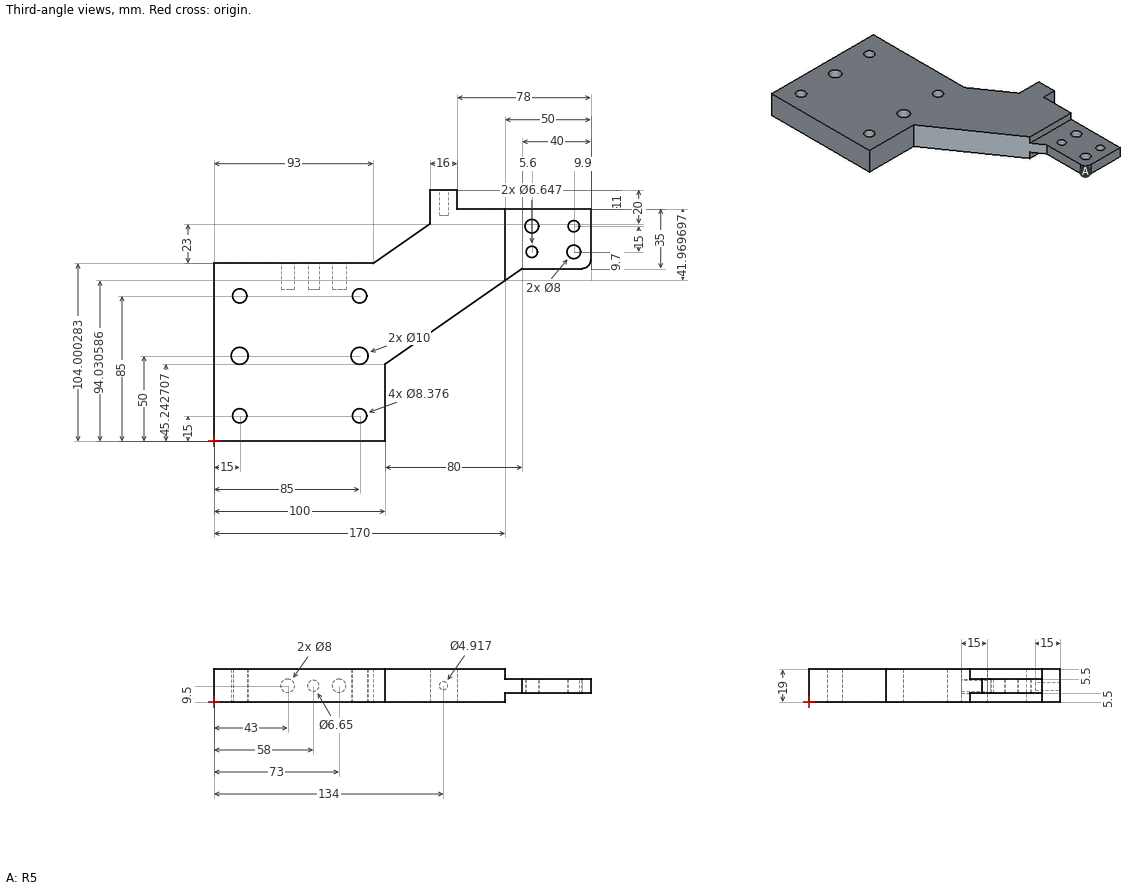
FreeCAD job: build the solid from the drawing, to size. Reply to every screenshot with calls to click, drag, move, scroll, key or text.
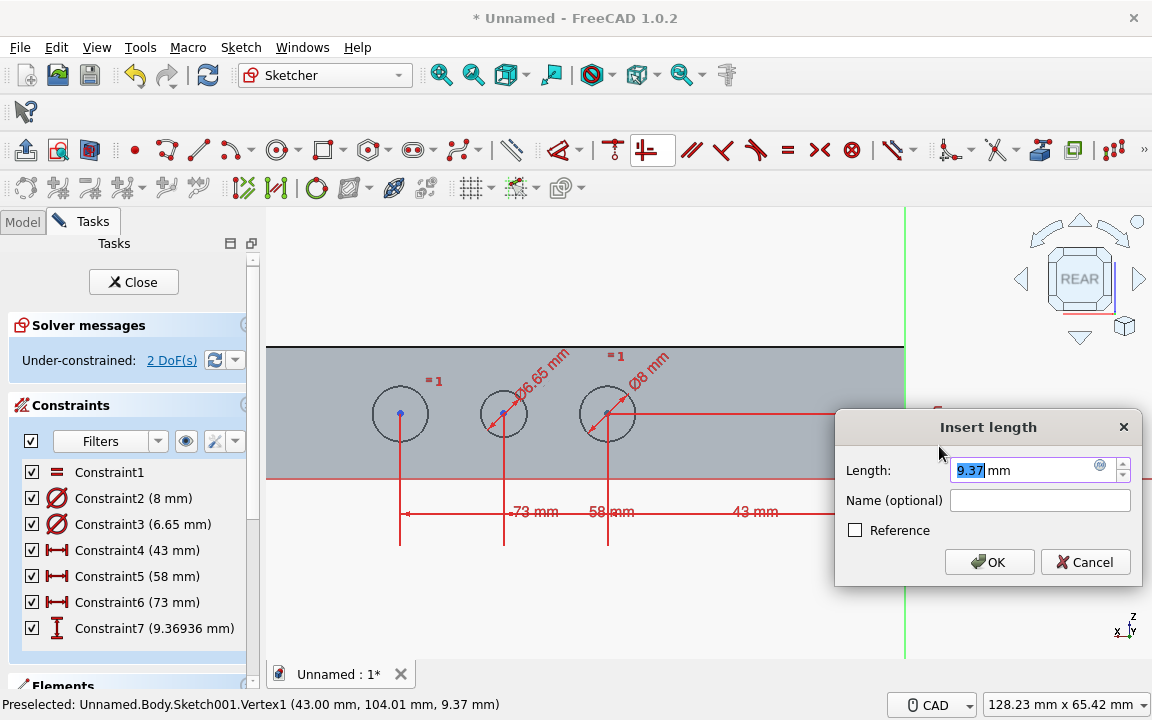
text(9.5)
key(Return)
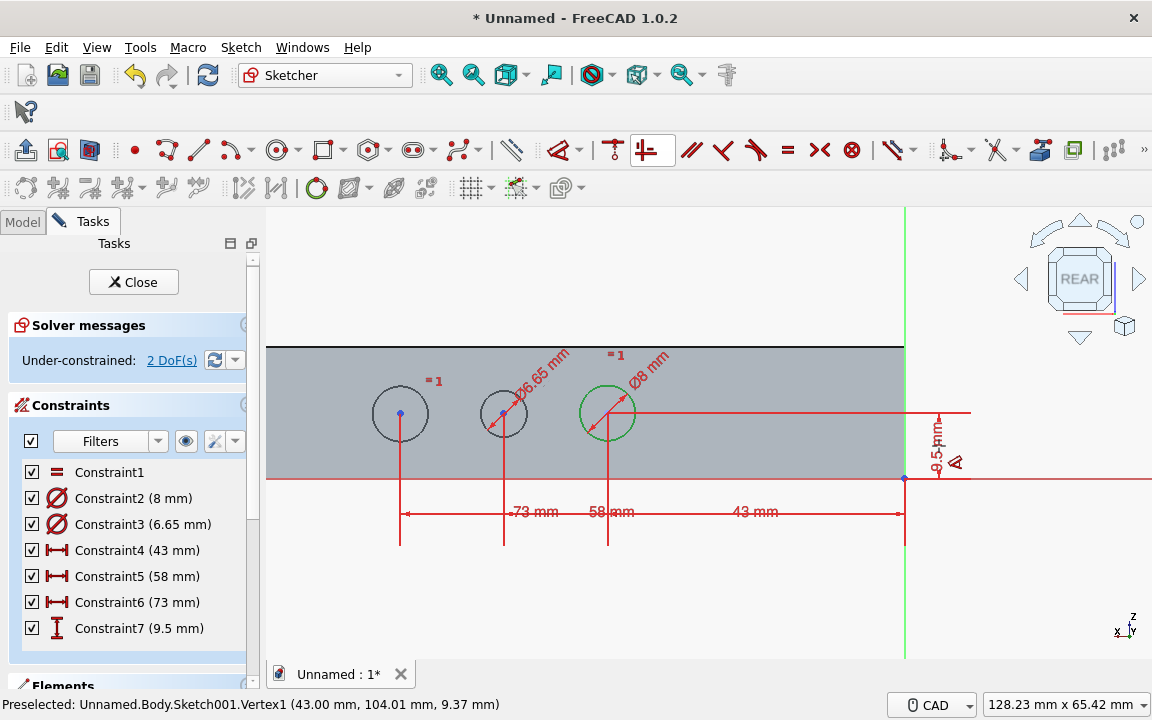
click(504, 414)
click(939, 424)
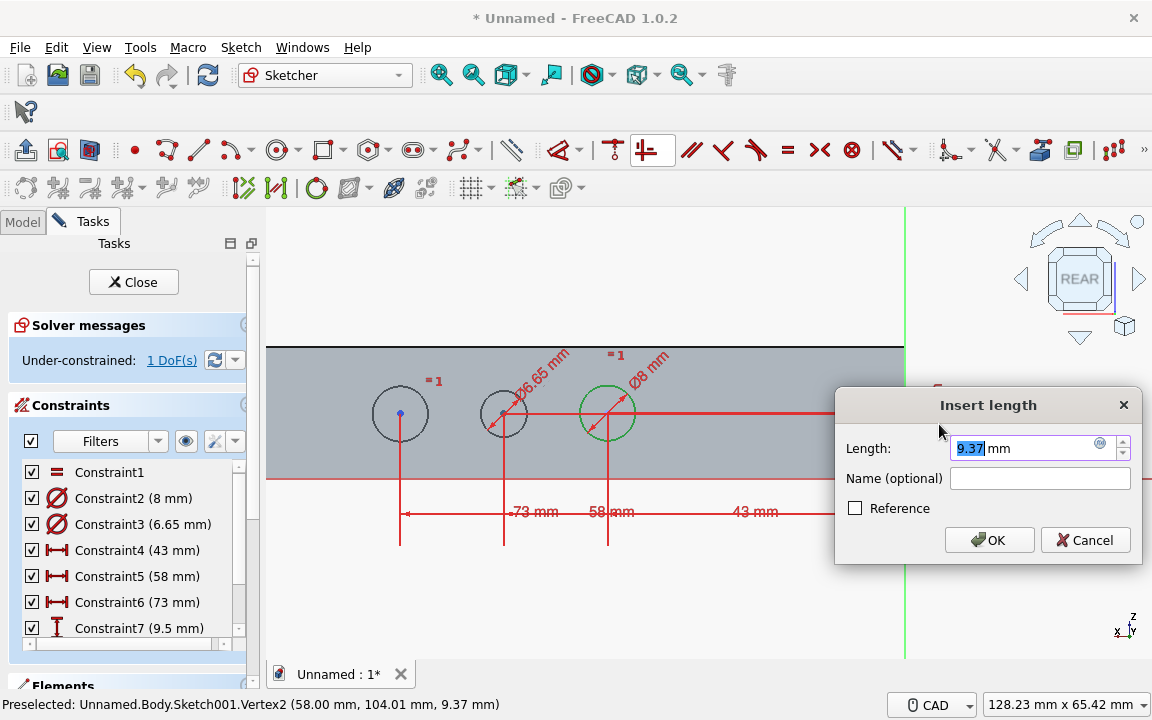
text(9.5)
key(Return)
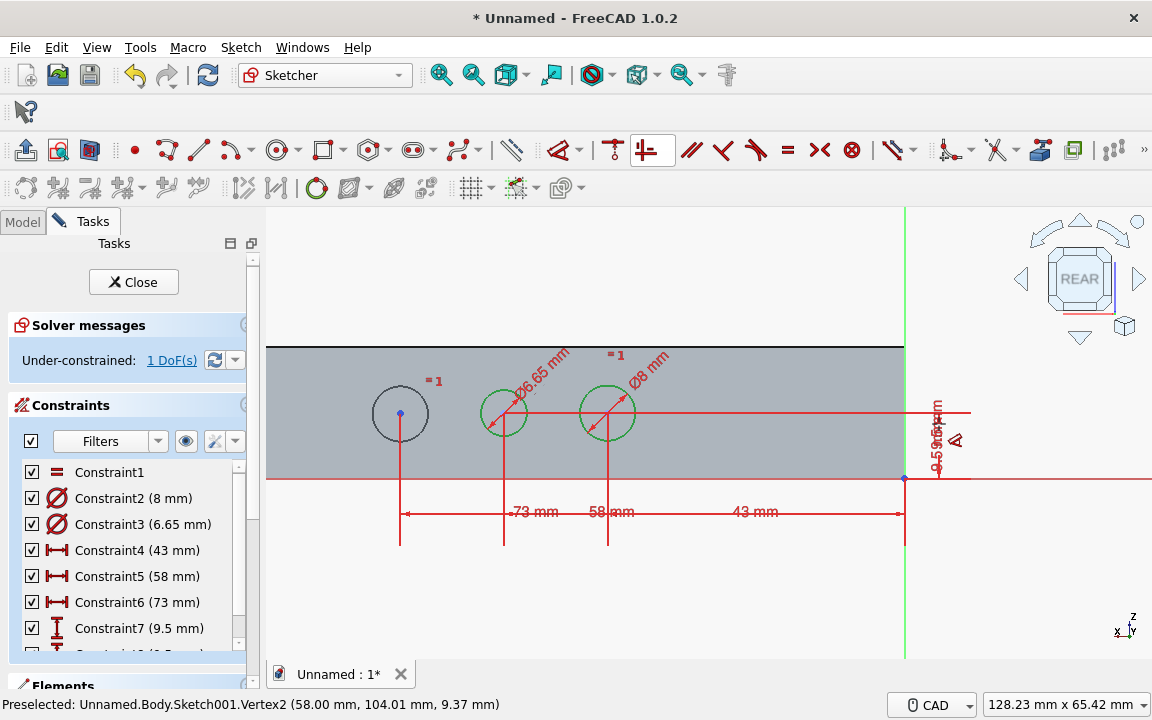
click(400, 414)
click(366, 446)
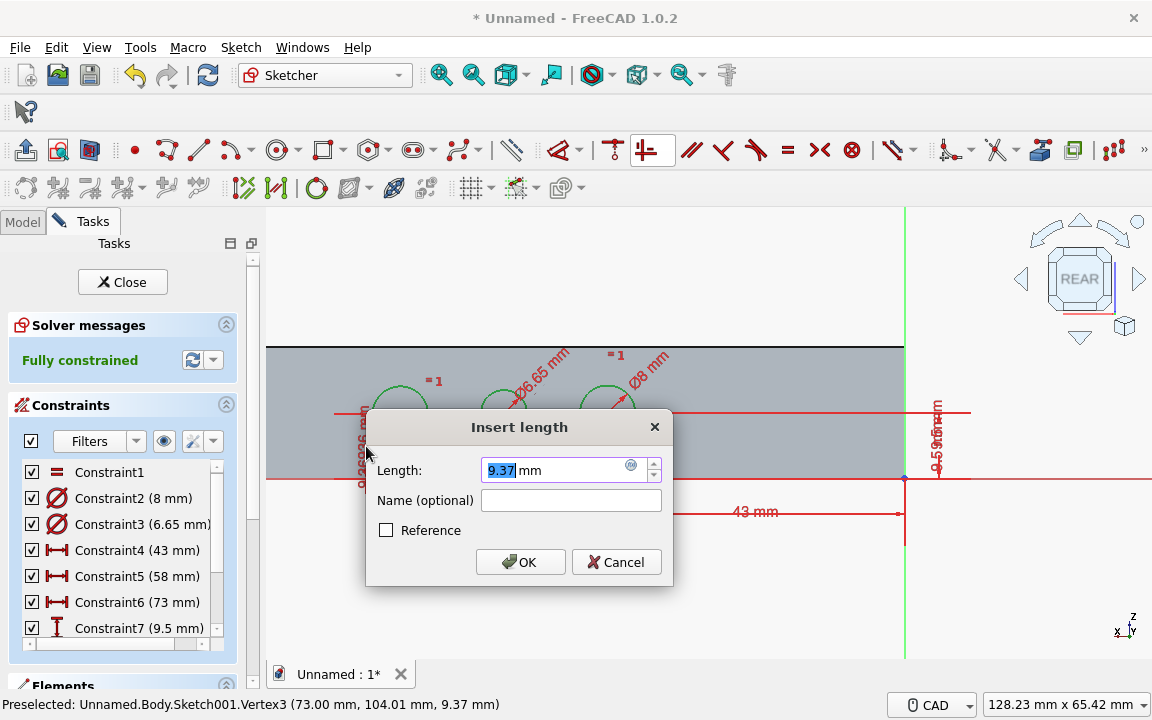
text(9.5)
key(Return)
key(Escape)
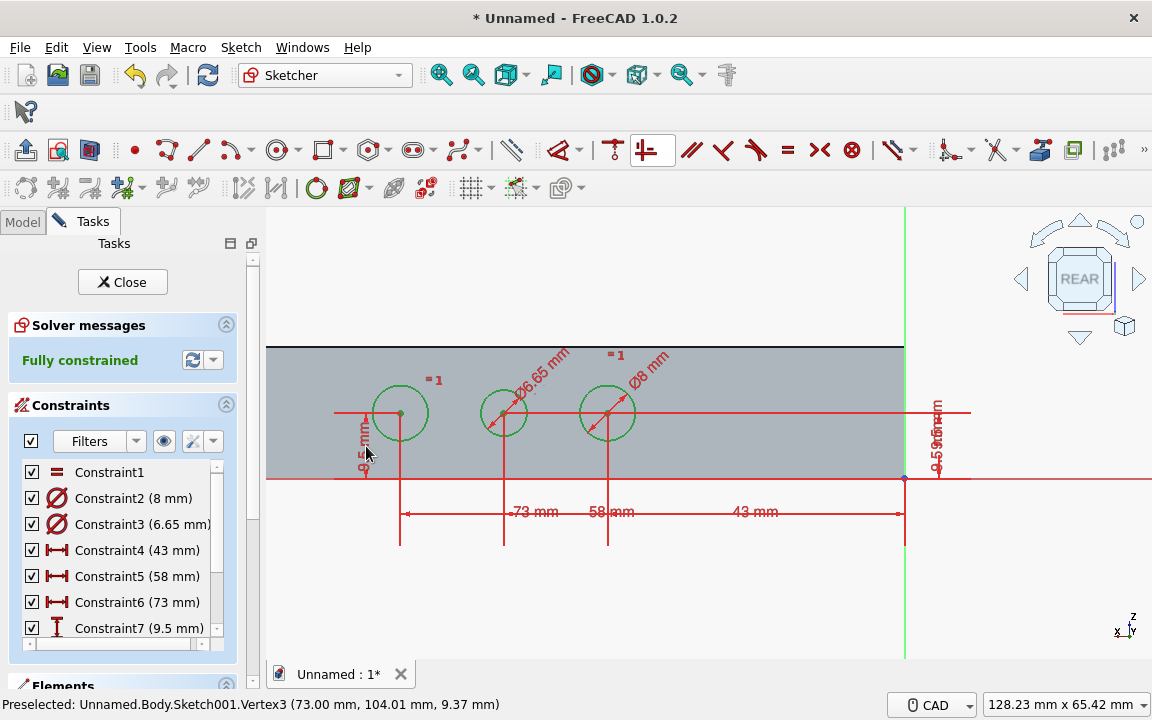
click(123, 282)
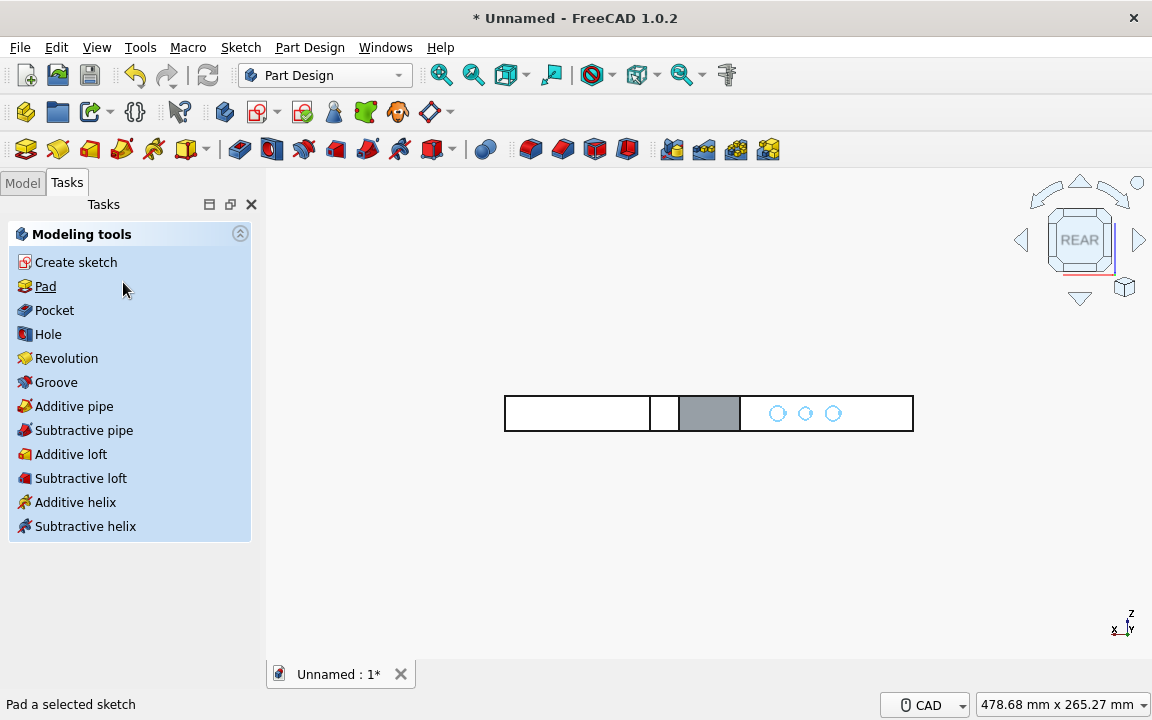
click(240, 150)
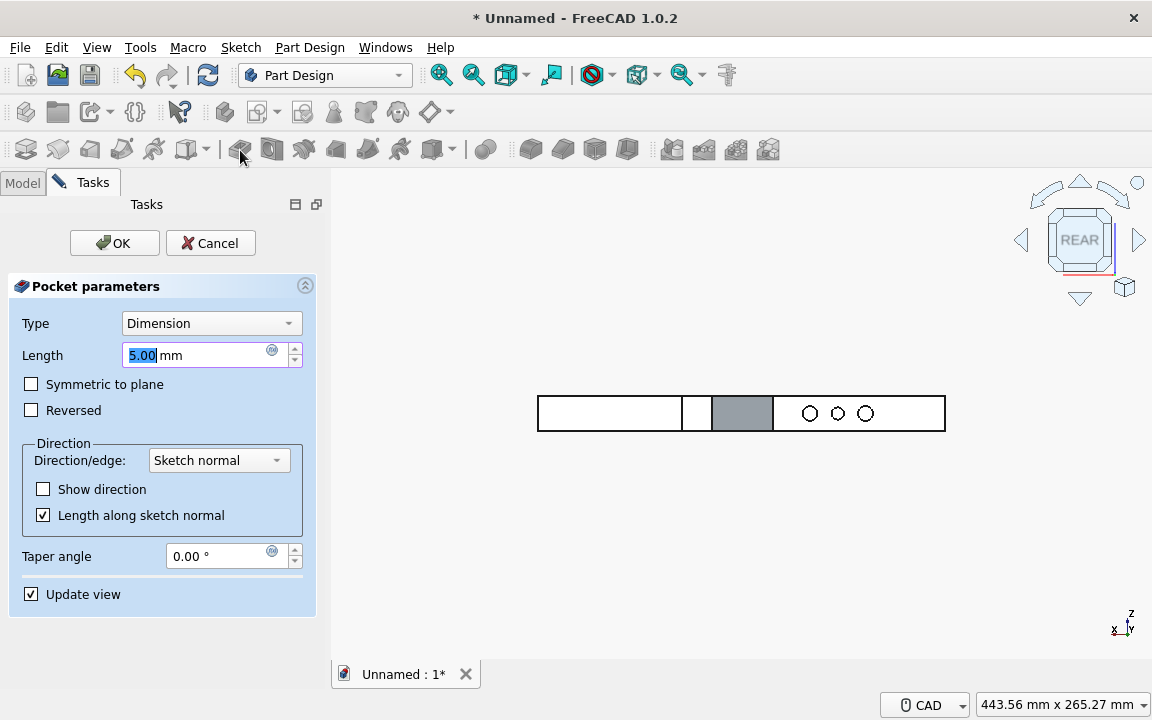
text(15)
key(Tab)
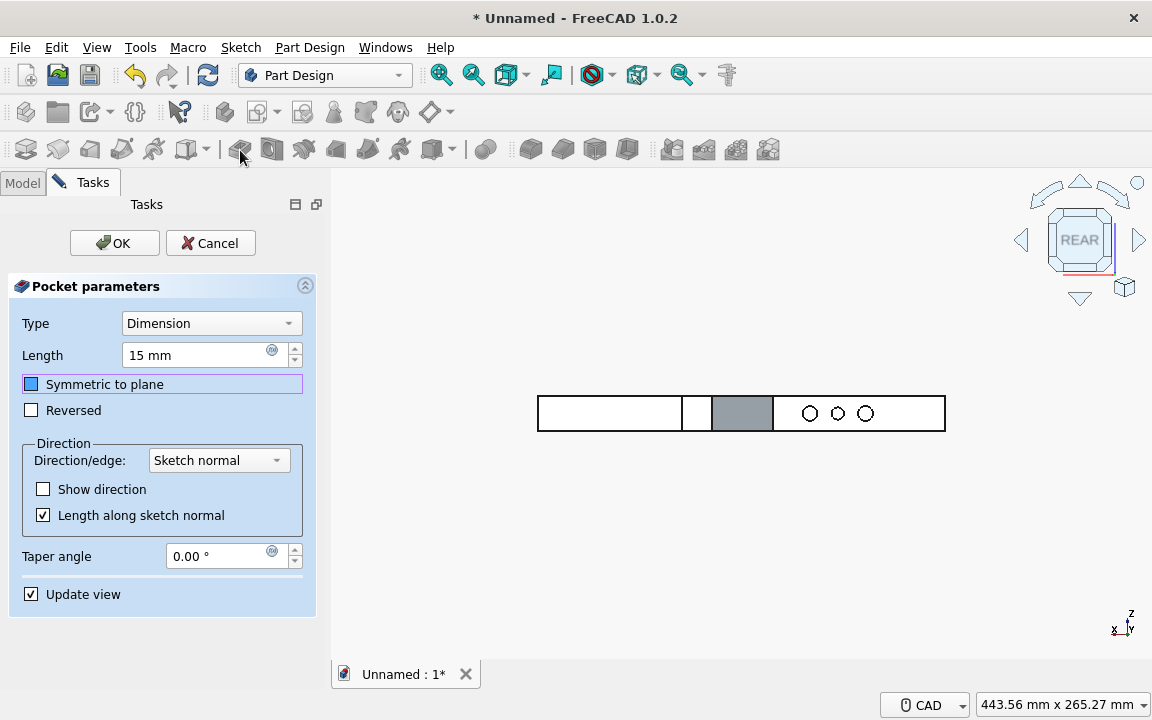
click(115, 243)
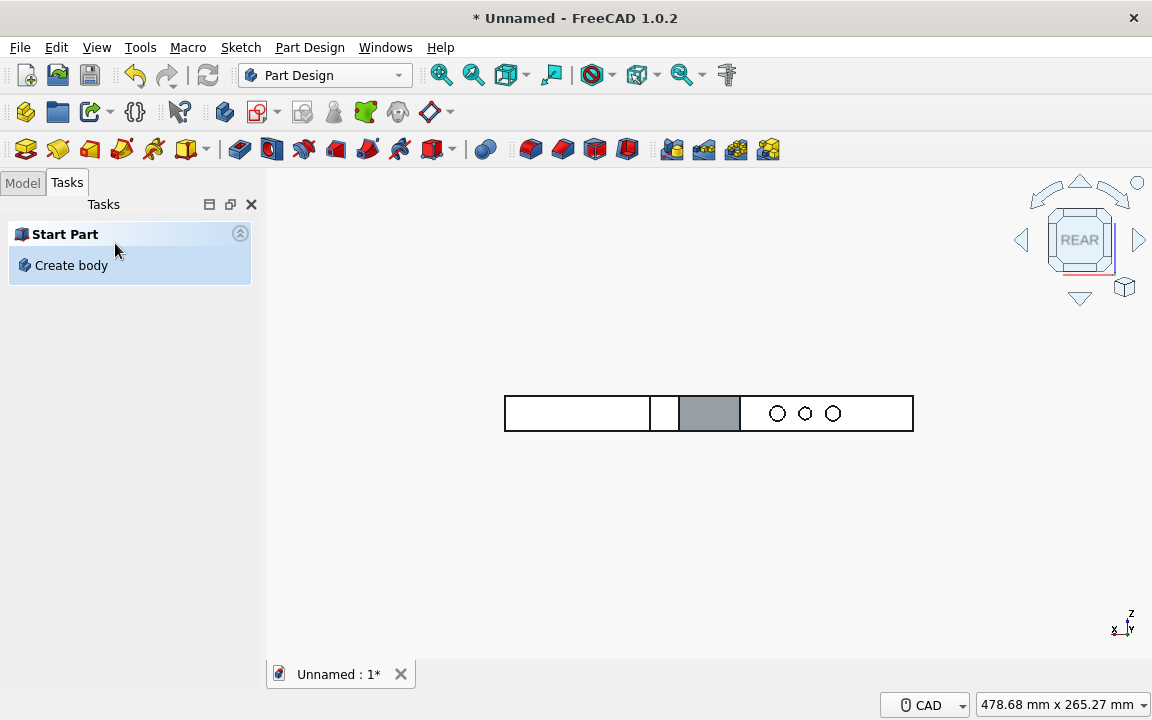
click(665, 413)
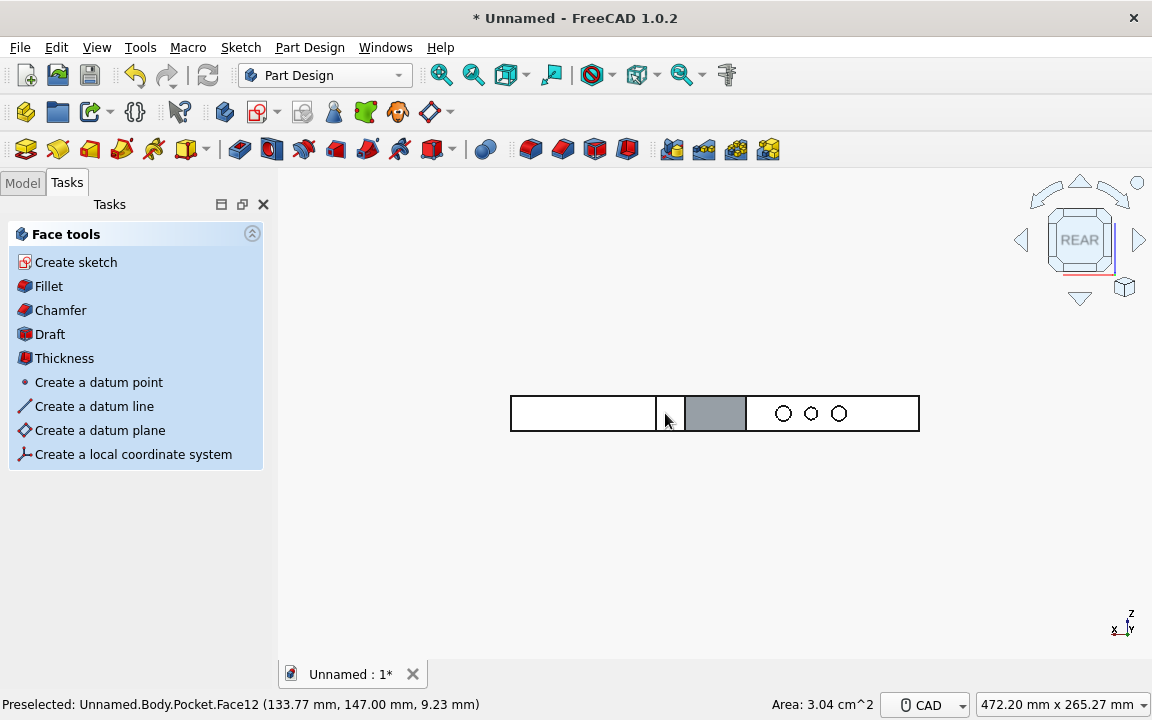
click(258, 112)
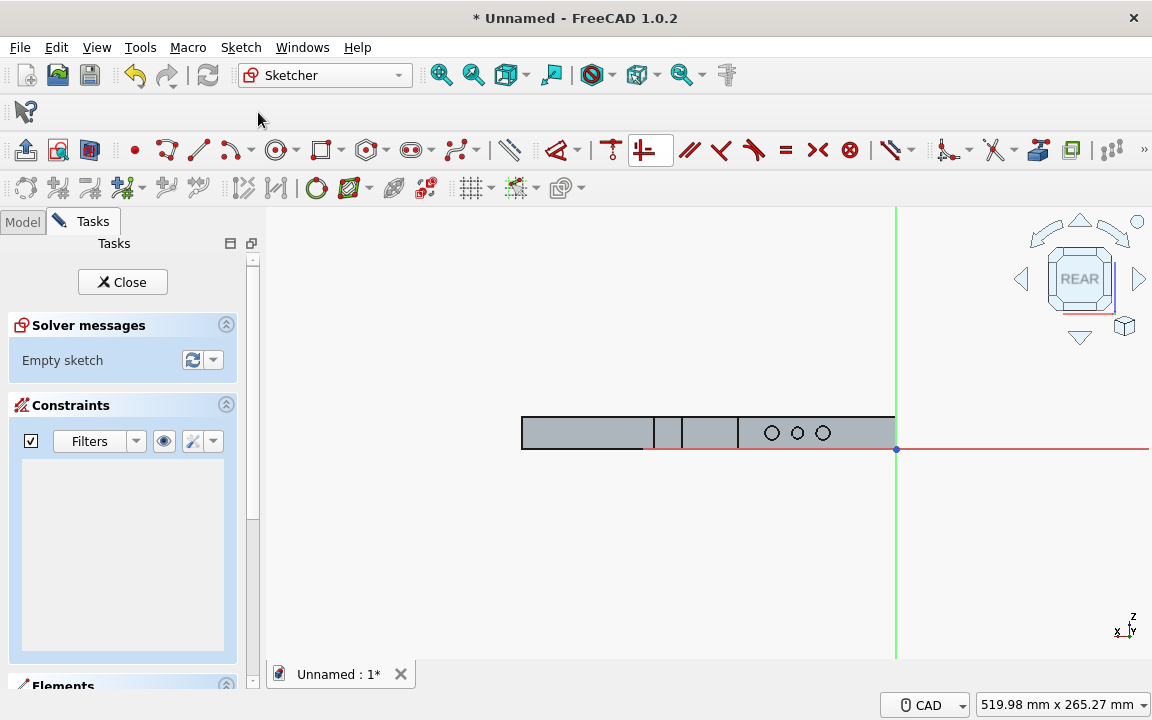
scroll(670, 433, up, 15)